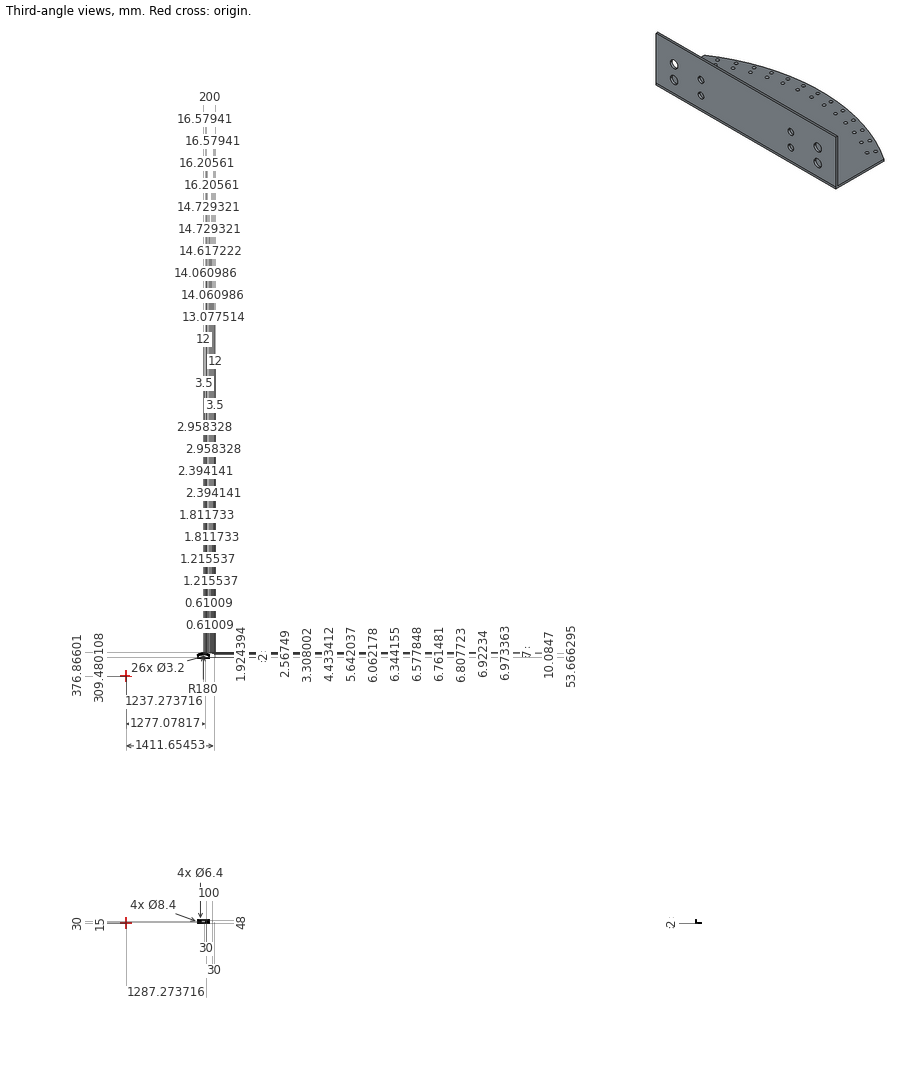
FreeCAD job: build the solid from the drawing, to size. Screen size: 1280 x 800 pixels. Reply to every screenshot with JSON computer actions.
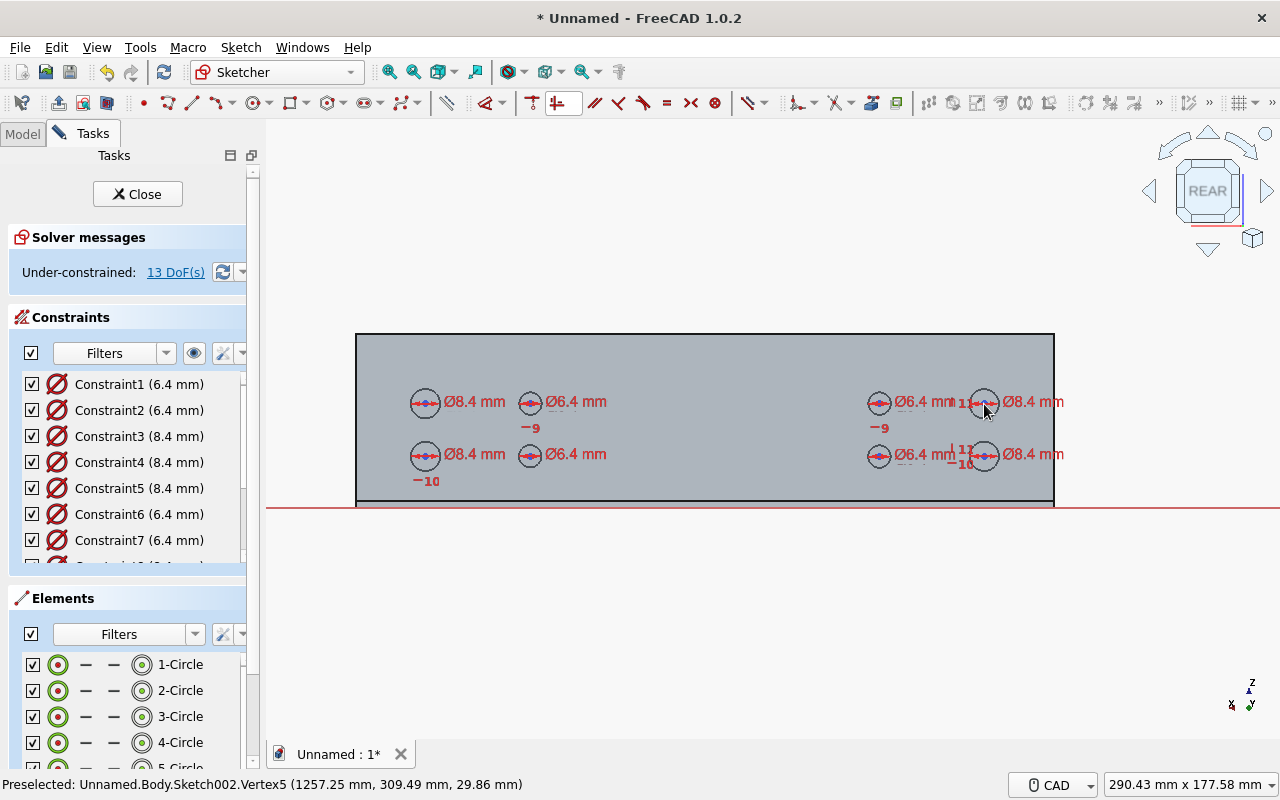
{"action": "left_click", "coordinate": [880, 404]}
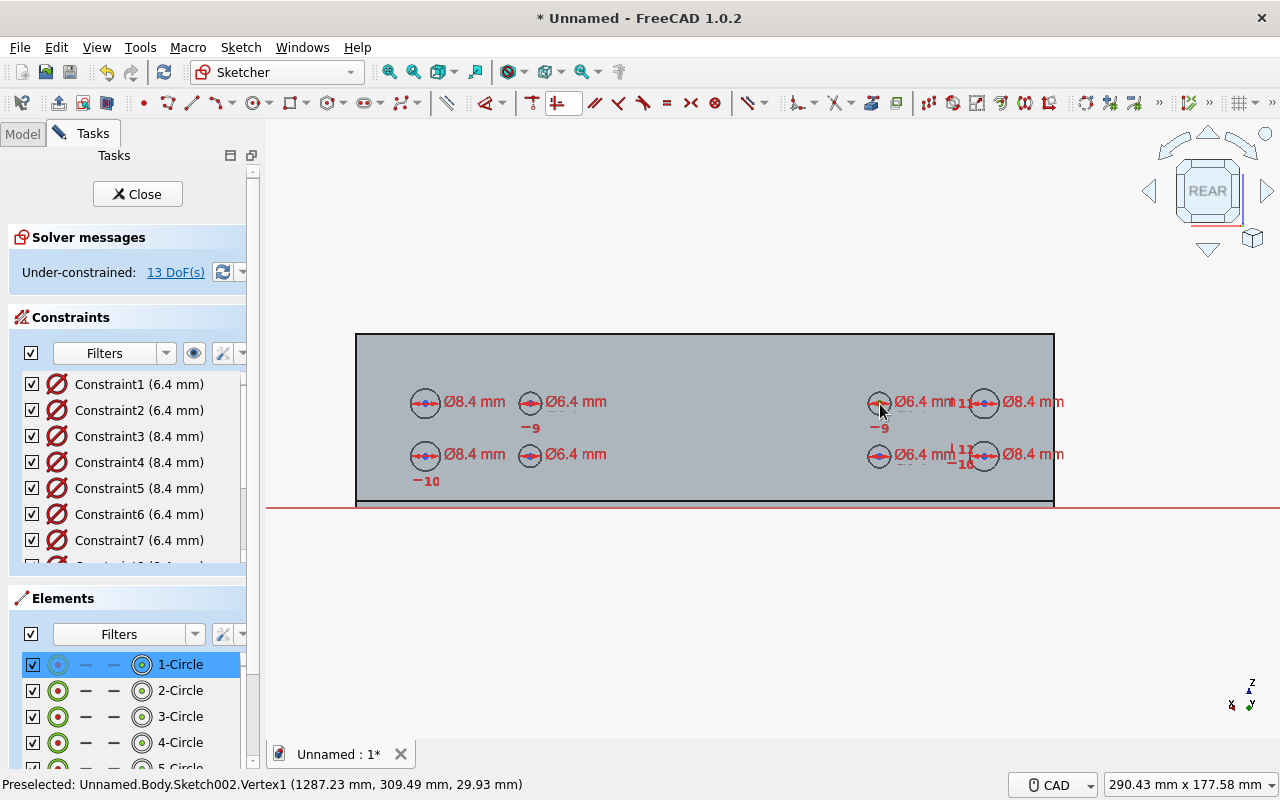
{"action": "left_click", "coordinate": [984, 404]}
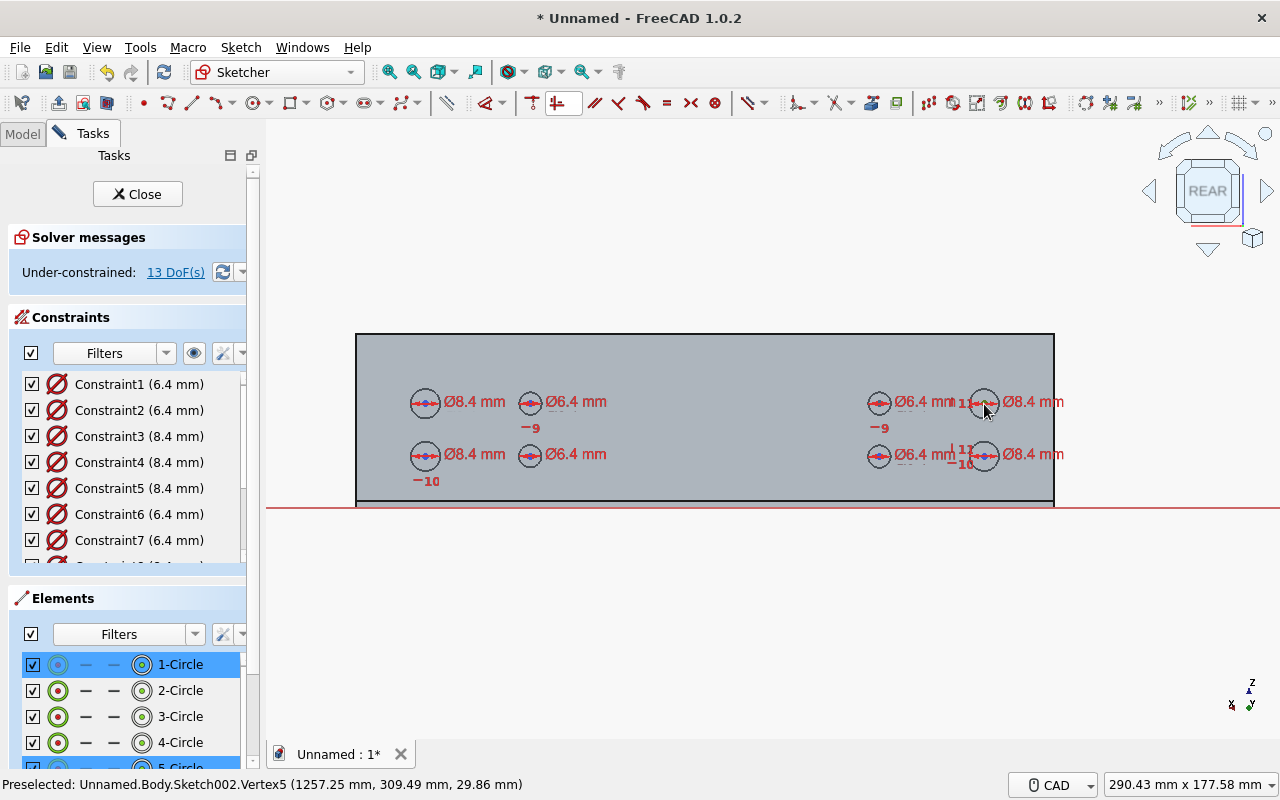
{"action": "left_click", "coordinate": [576, 104]}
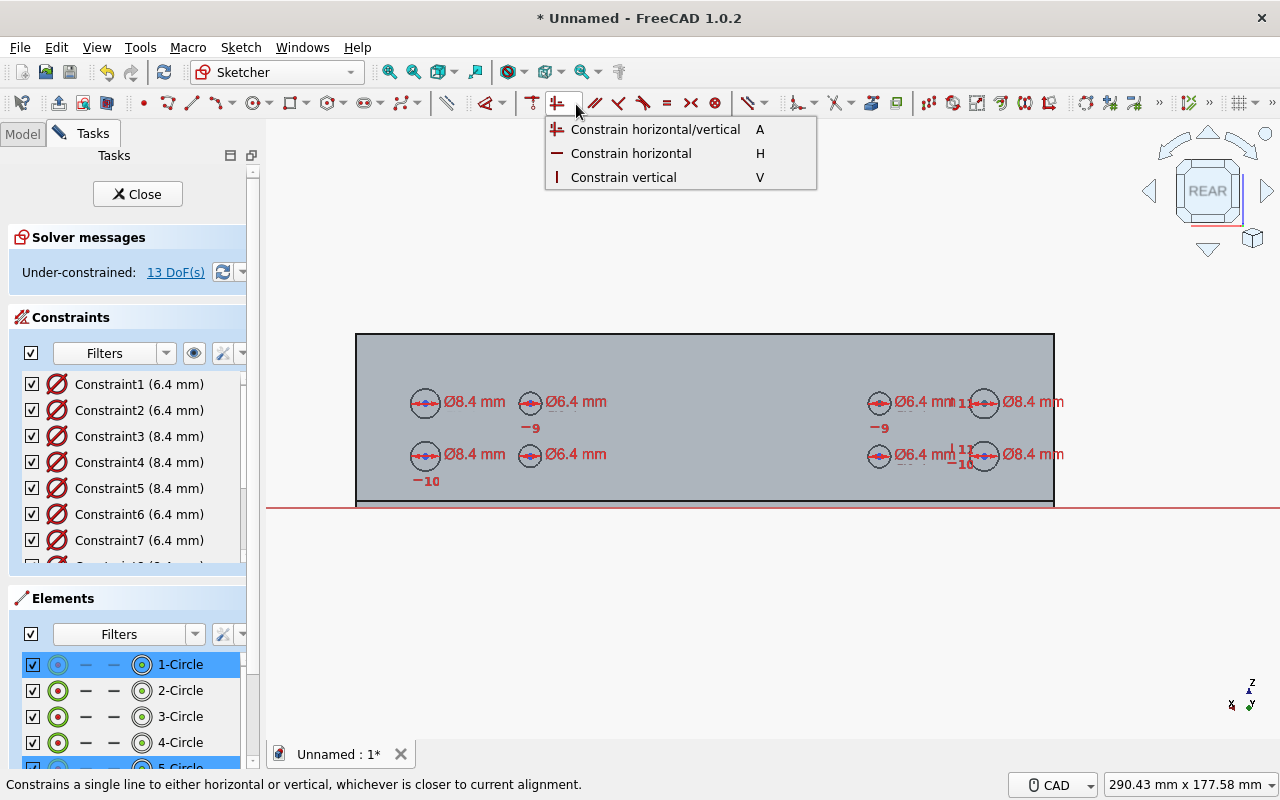
{"action": "left_click", "coordinate": [681, 153]}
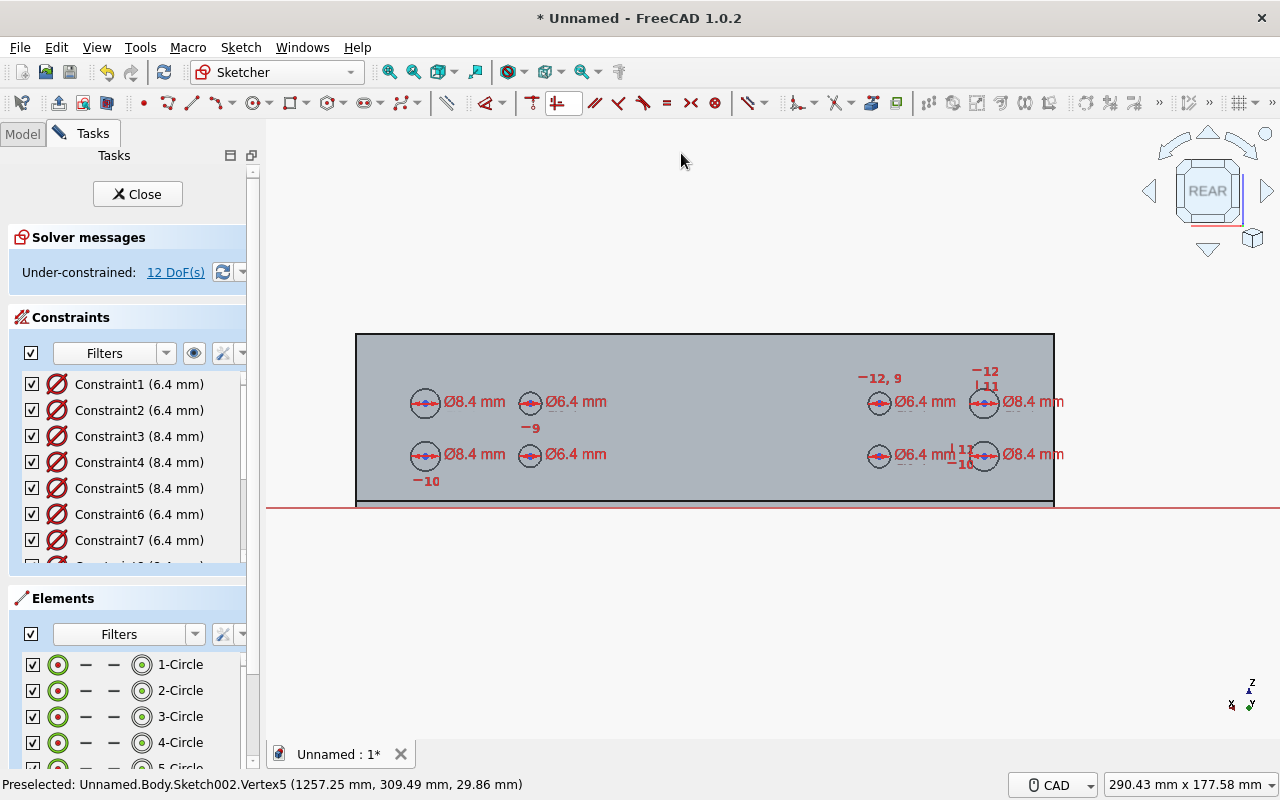
{"action": "left_click", "coordinate": [880, 404]}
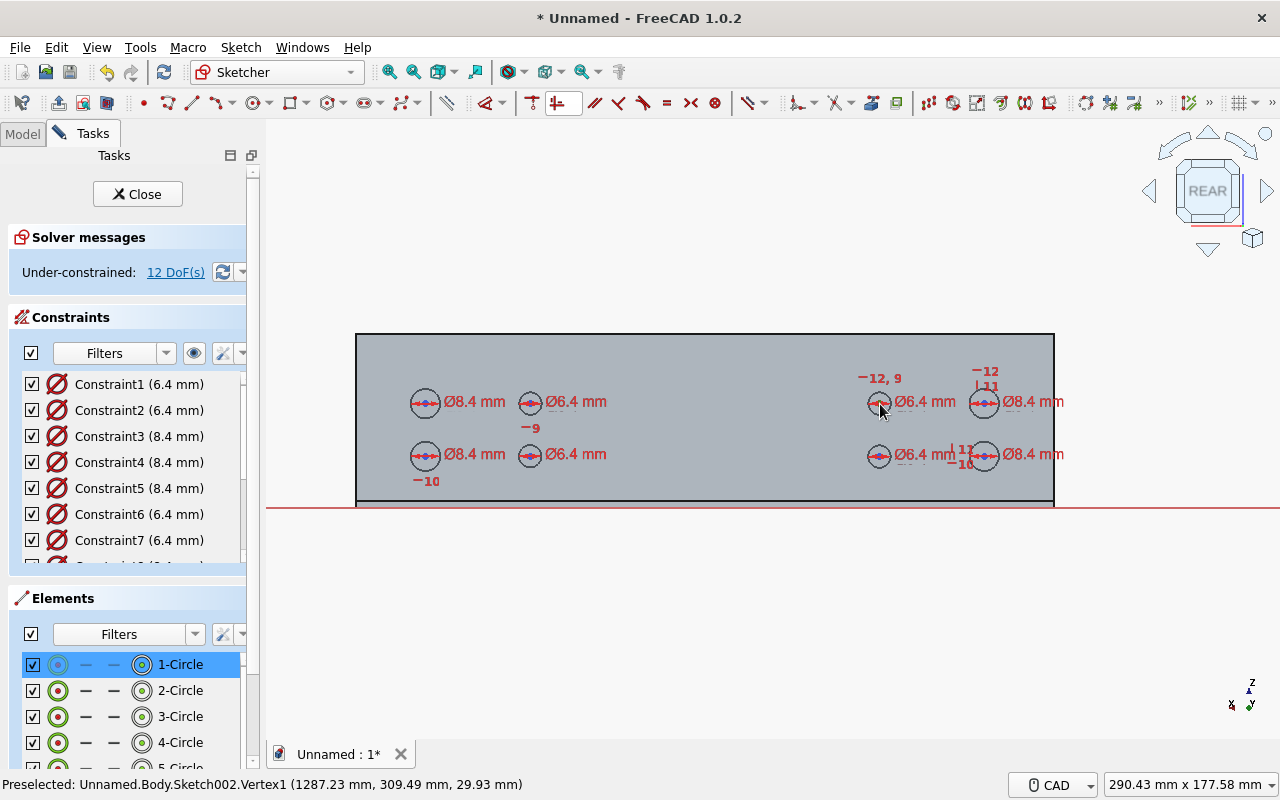
{"action": "left_click", "coordinate": [879, 457]}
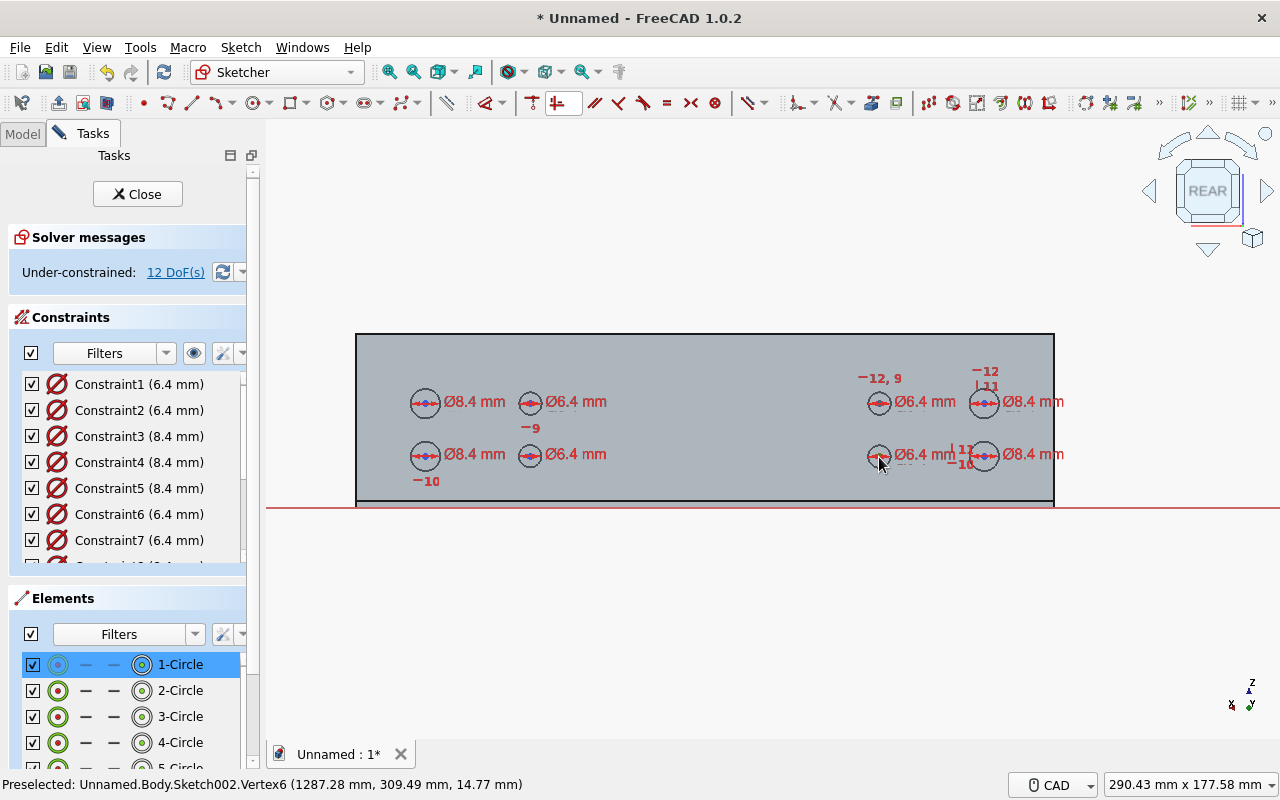
{"action": "key", "text": "v"}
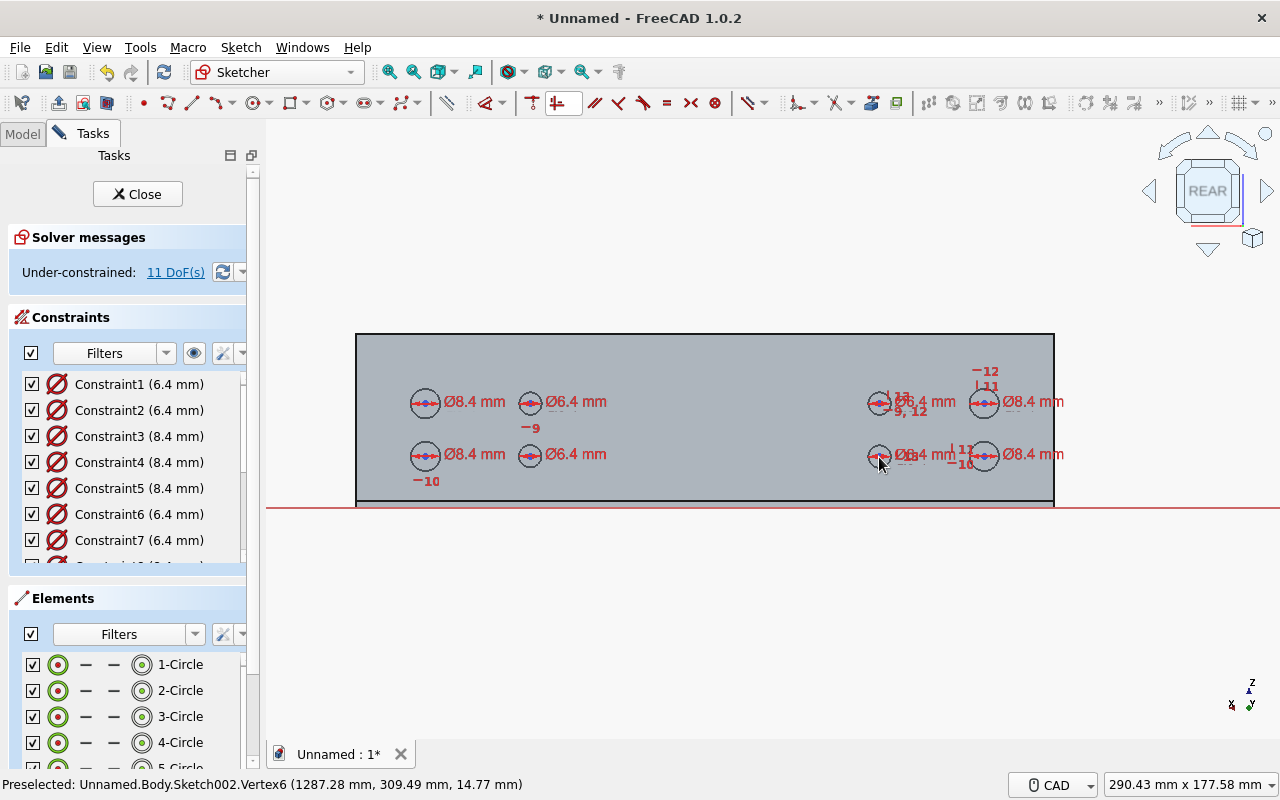
{"action": "left_click", "coordinate": [984, 456]}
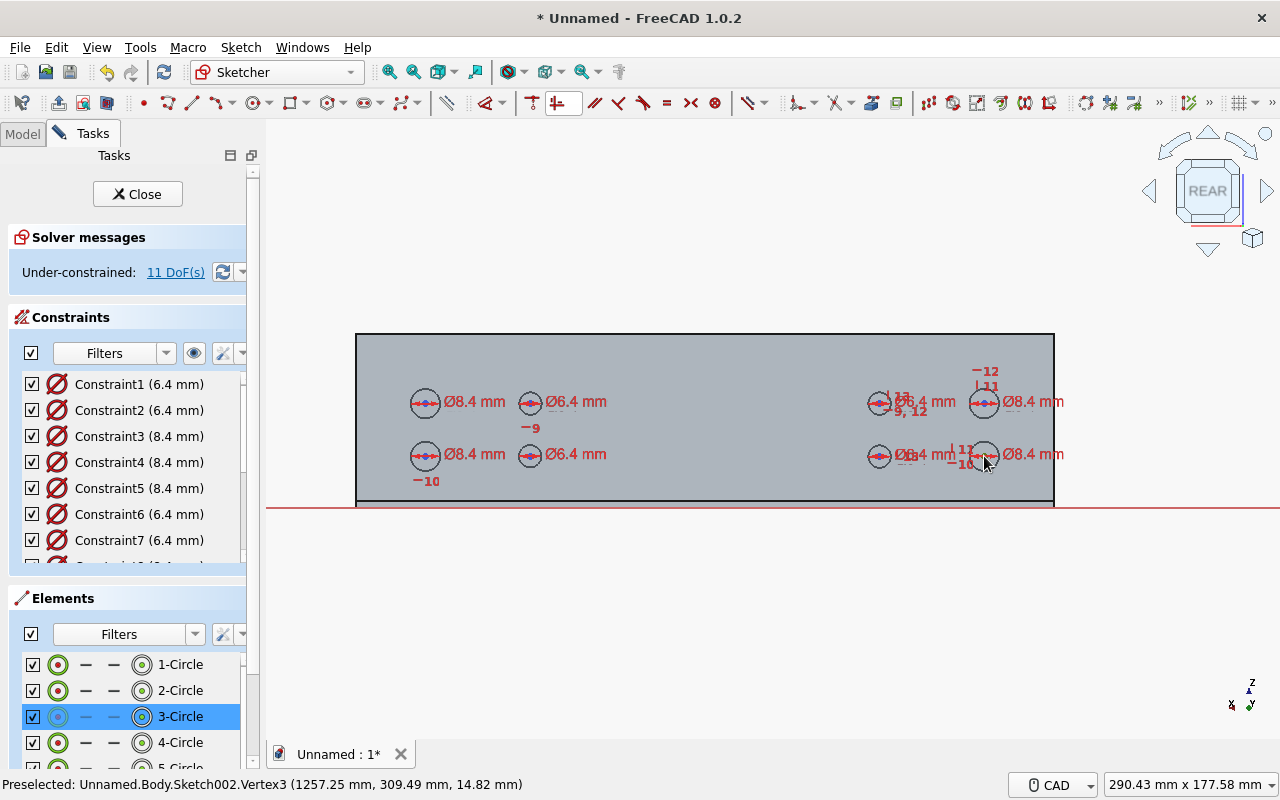
{"action": "left_click", "coordinate": [880, 457]}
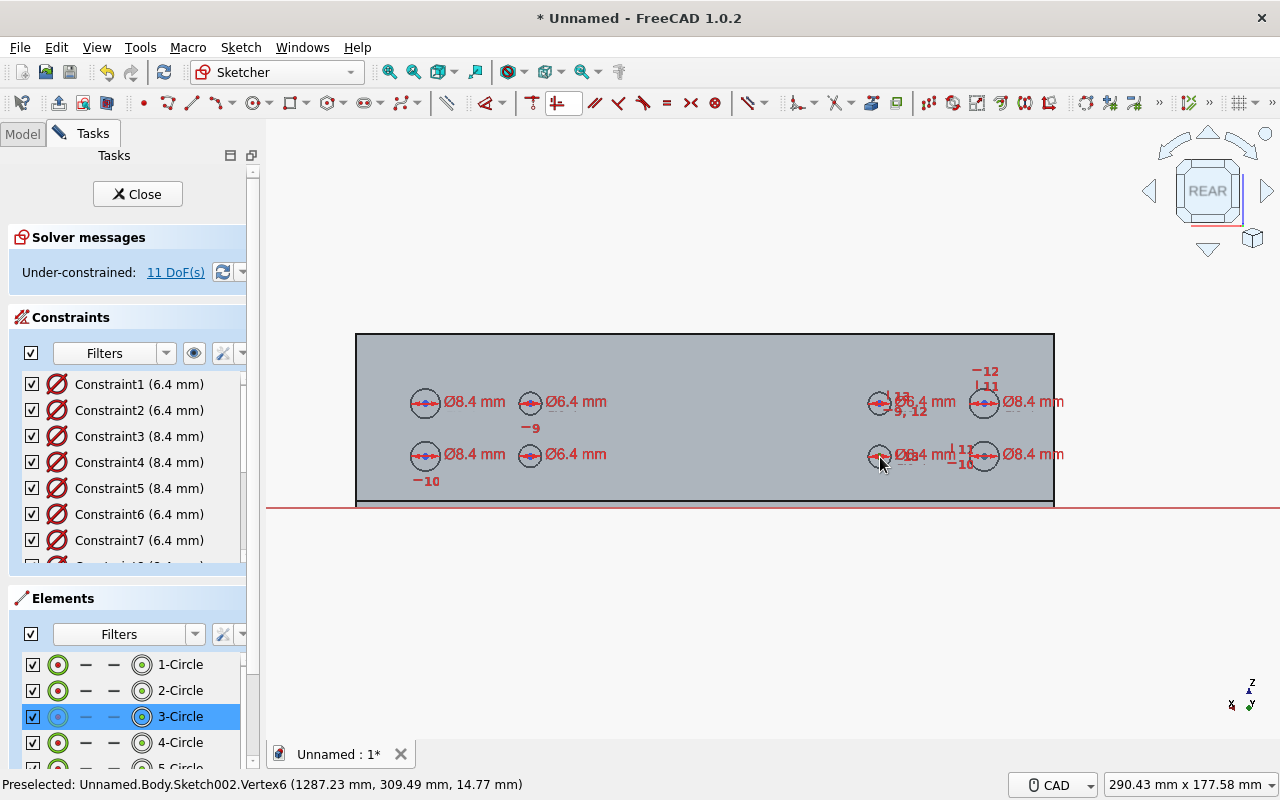
{"action": "key", "text": "h"}